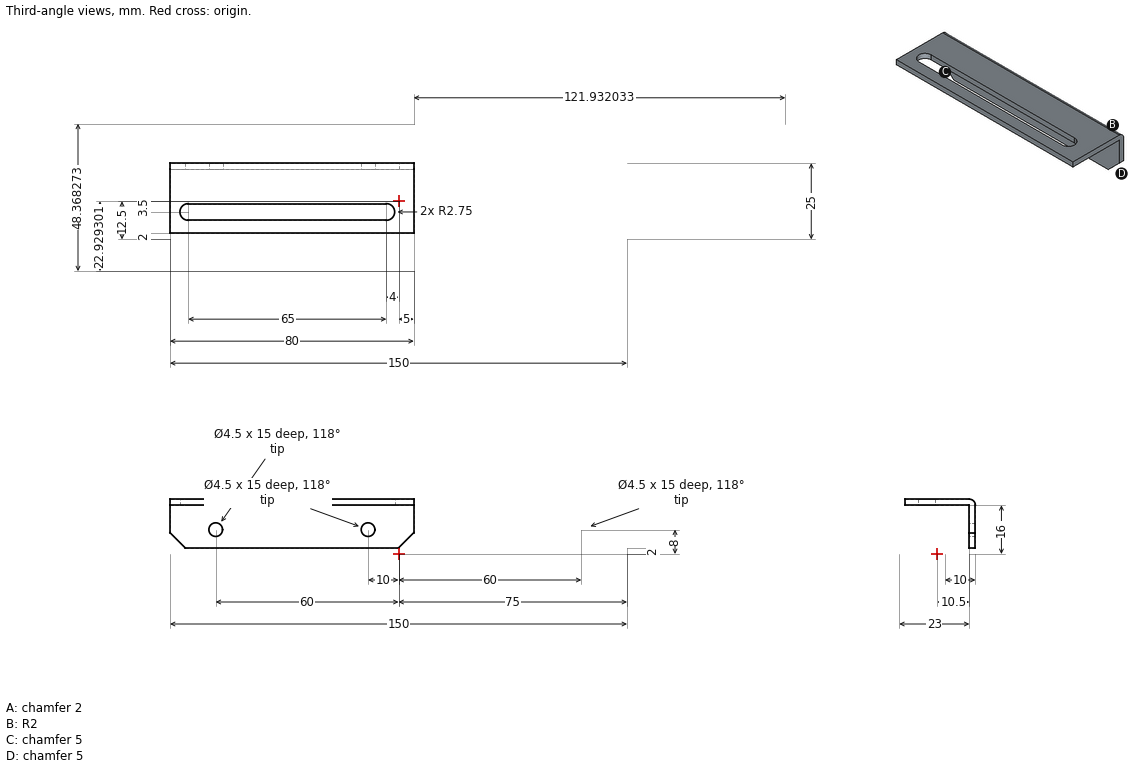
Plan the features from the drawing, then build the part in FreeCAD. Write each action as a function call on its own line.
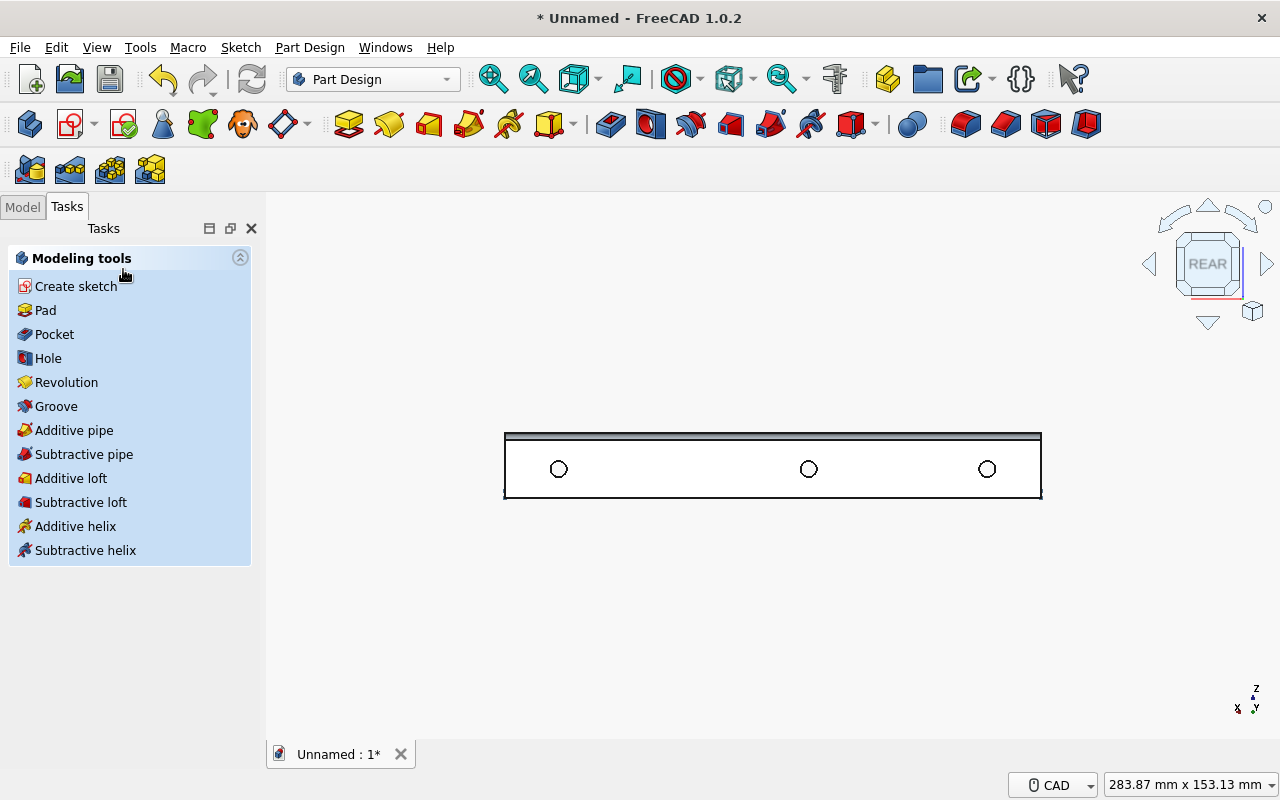
click(612, 124)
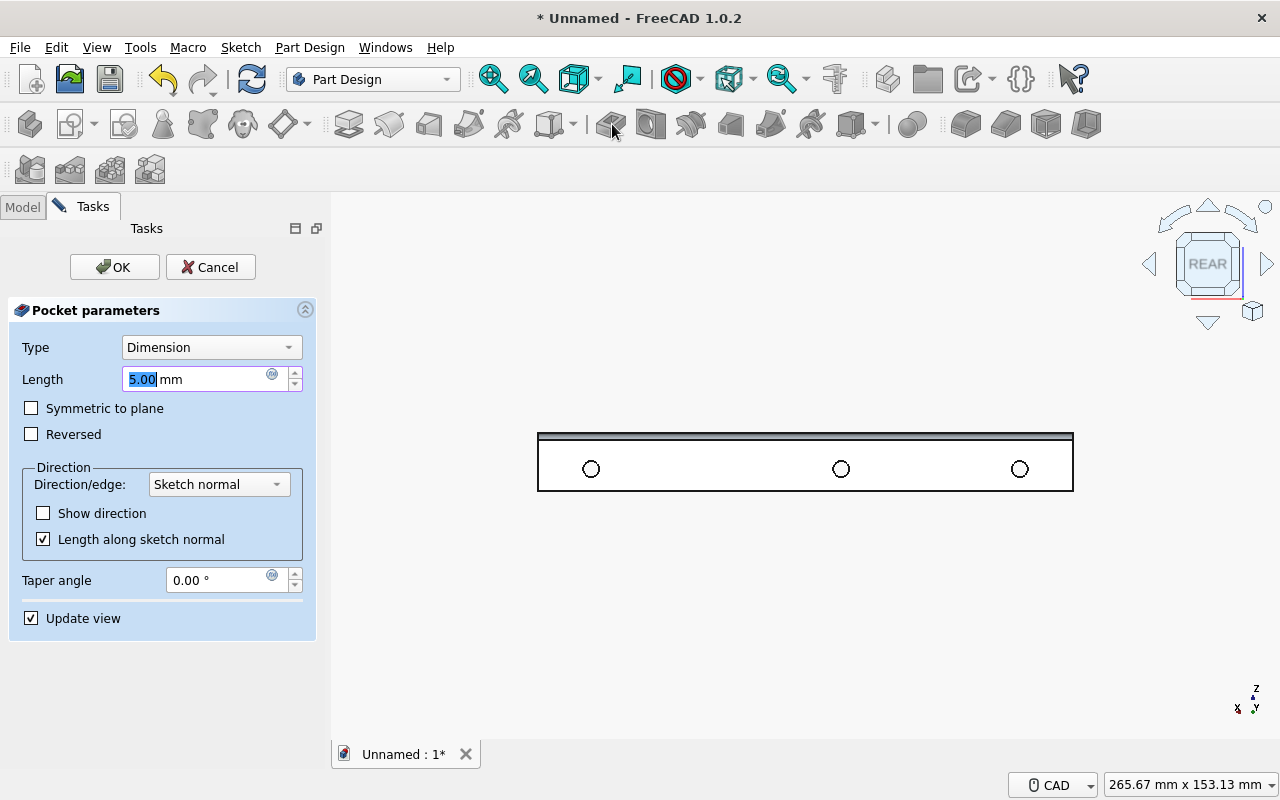
text(10)
key(Tab)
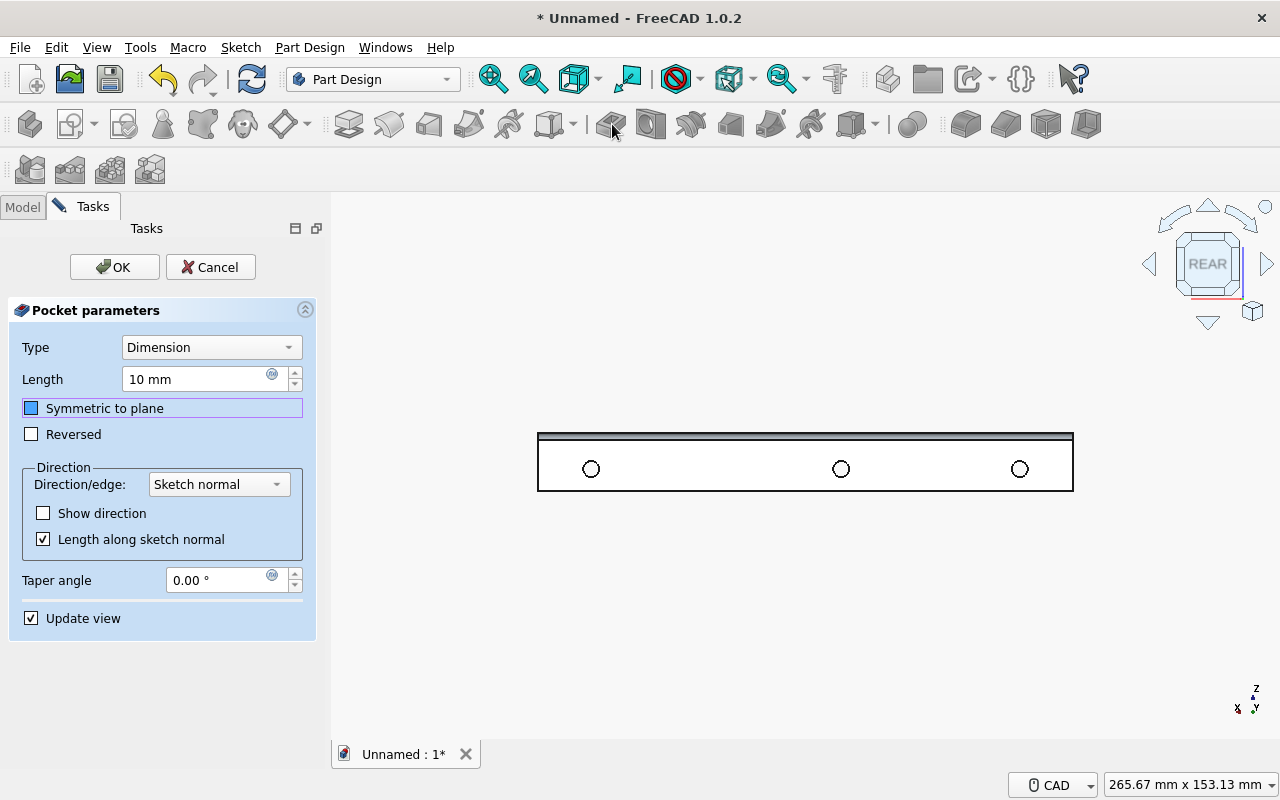
click(115, 267)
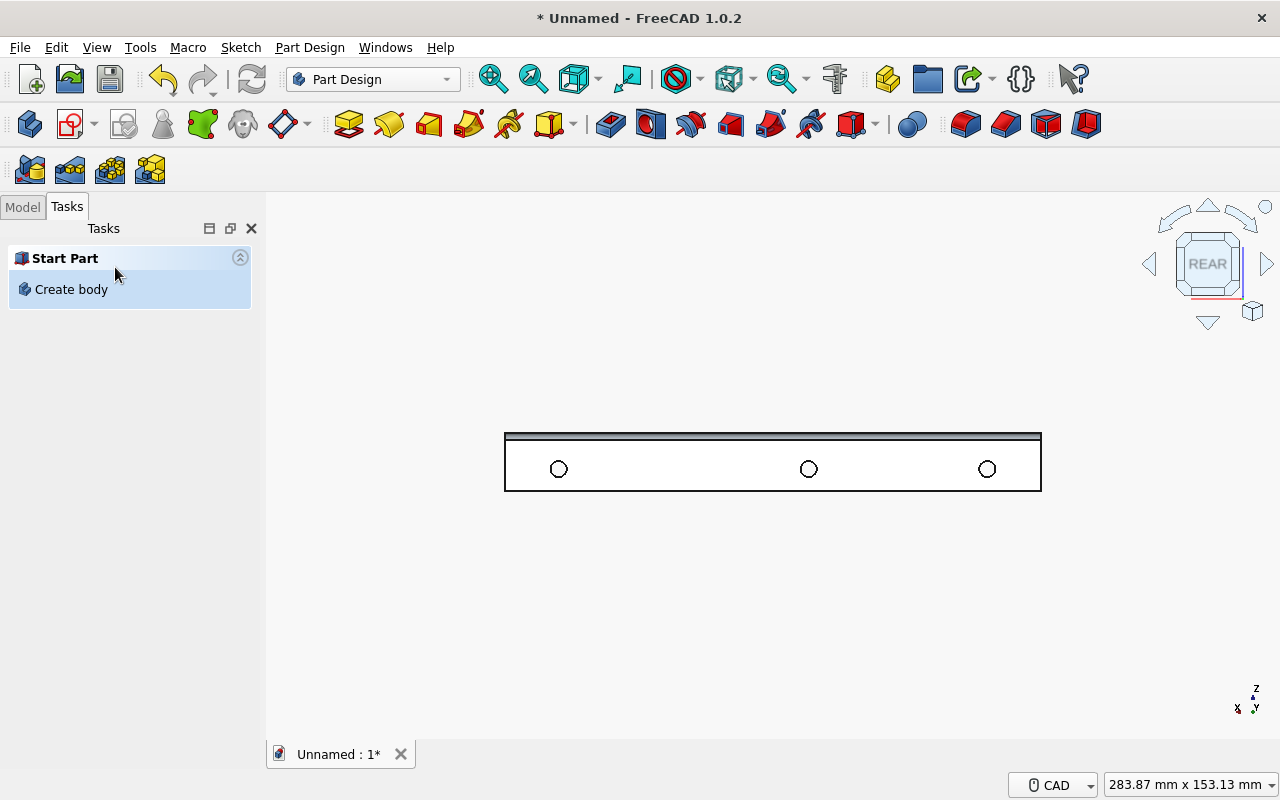
scroll(505, 490, up, 9)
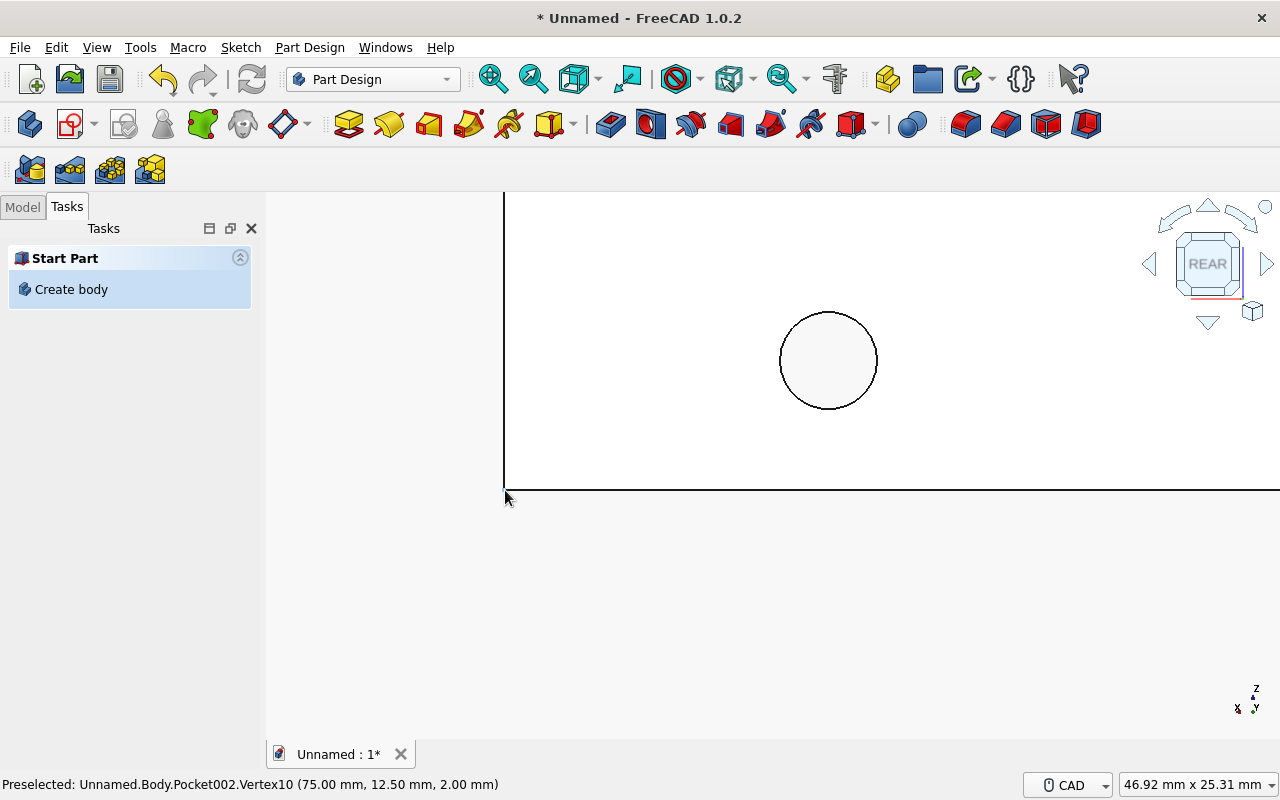
click(494, 80)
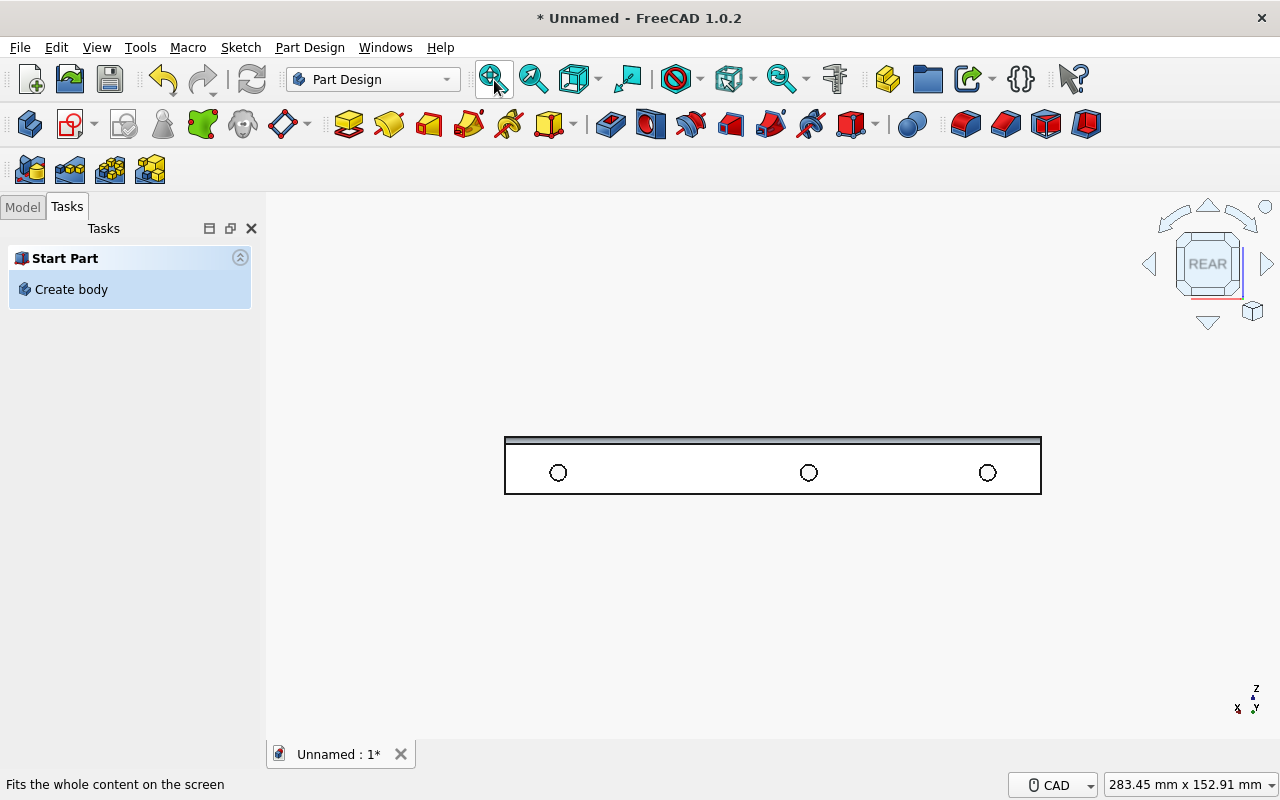
key(0)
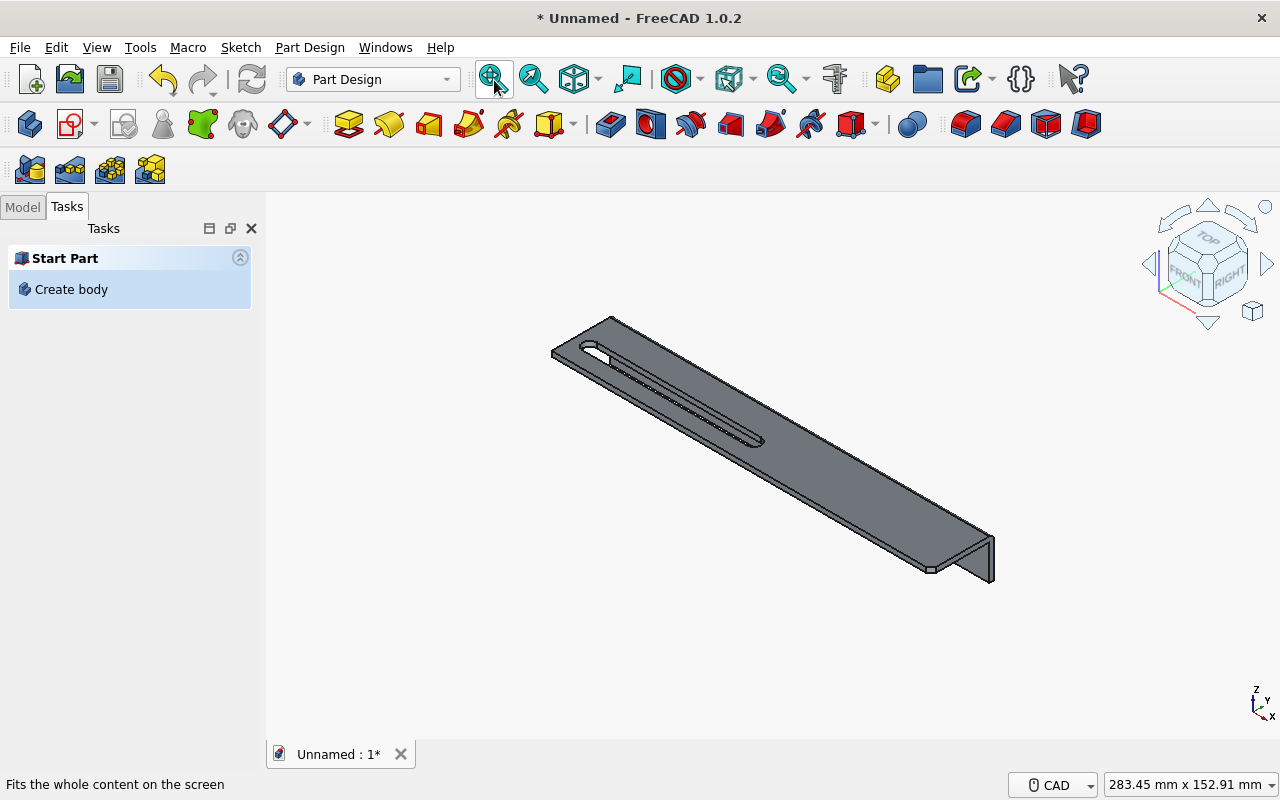
scroll(992, 581, up, 9)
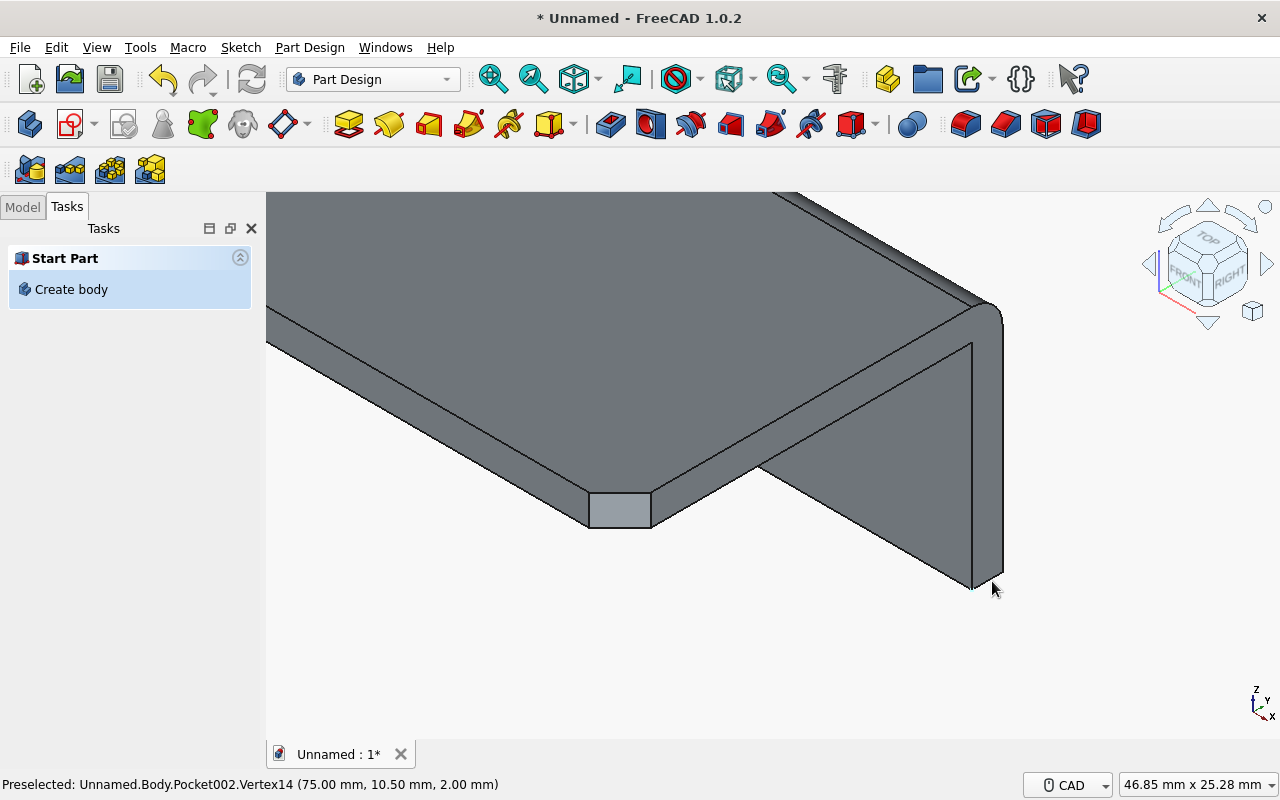
click(494, 80)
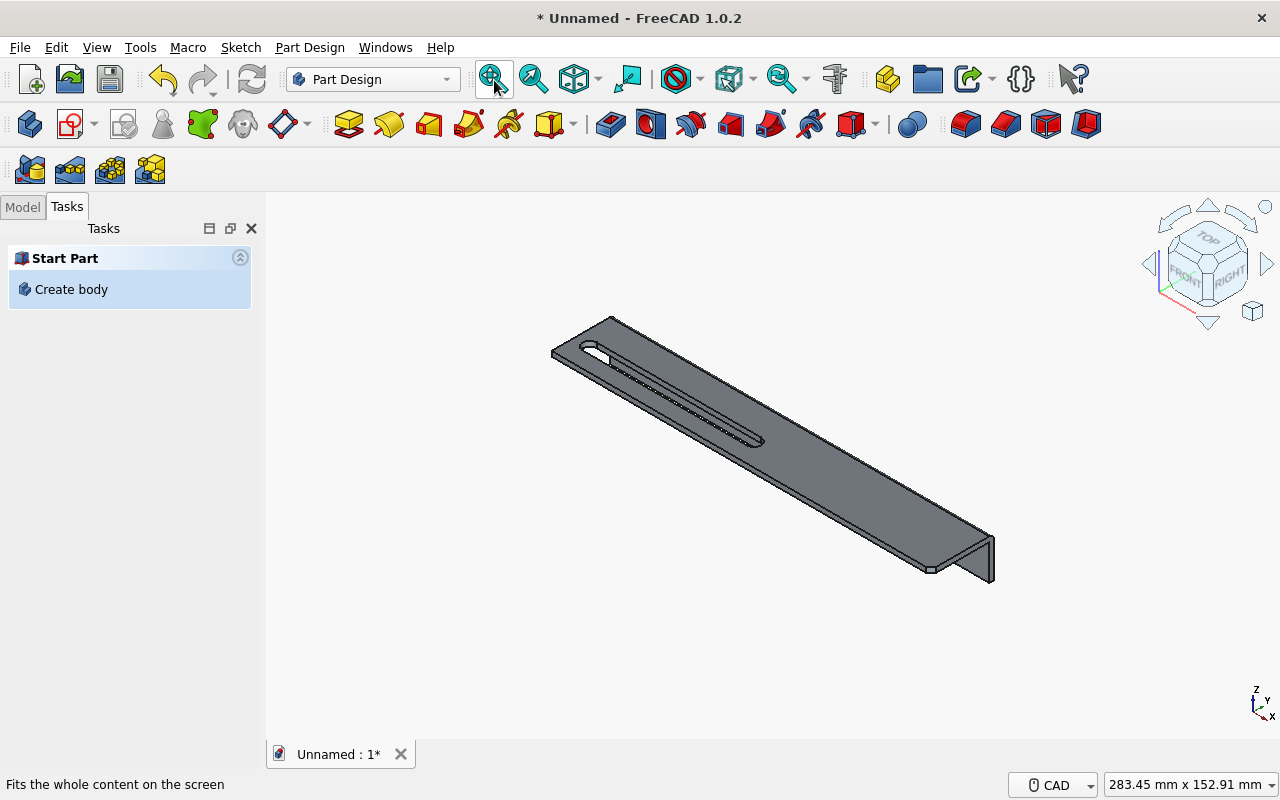
key(2)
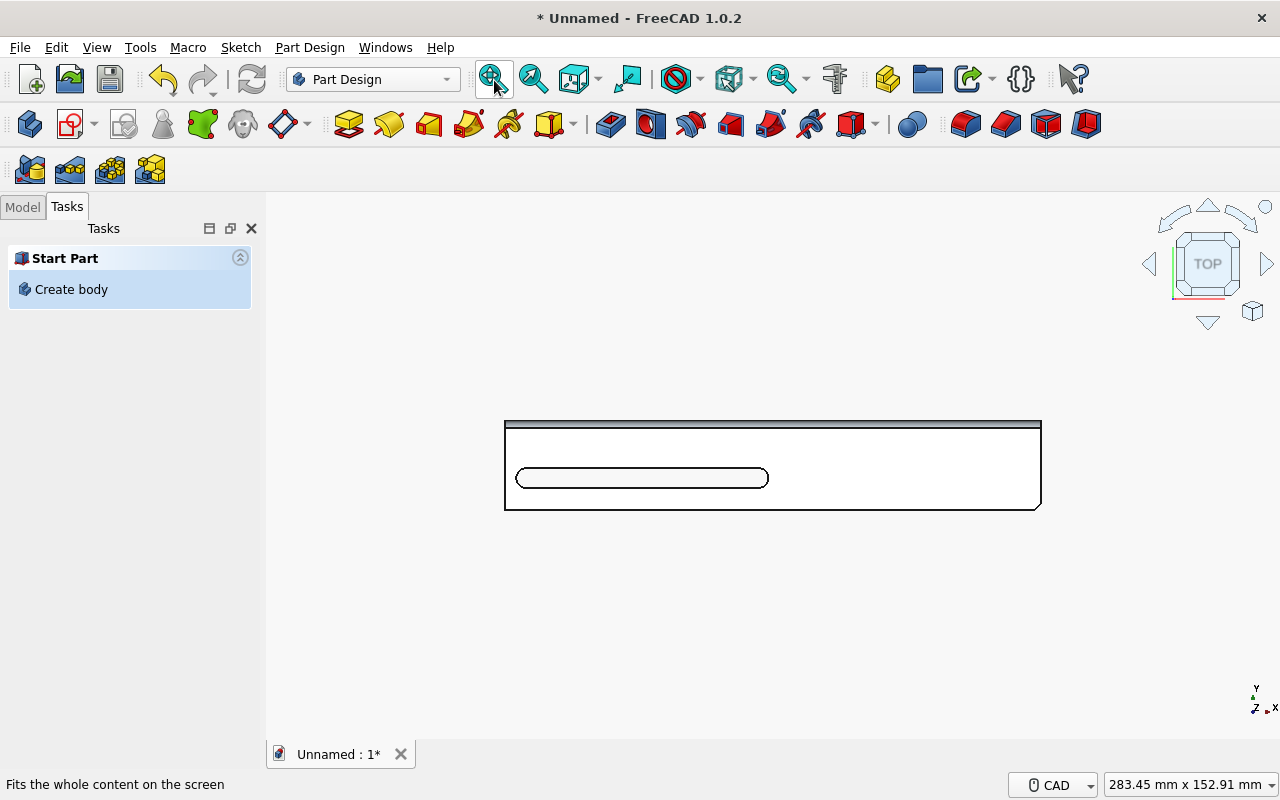
scroll(1041, 423, up, 9)